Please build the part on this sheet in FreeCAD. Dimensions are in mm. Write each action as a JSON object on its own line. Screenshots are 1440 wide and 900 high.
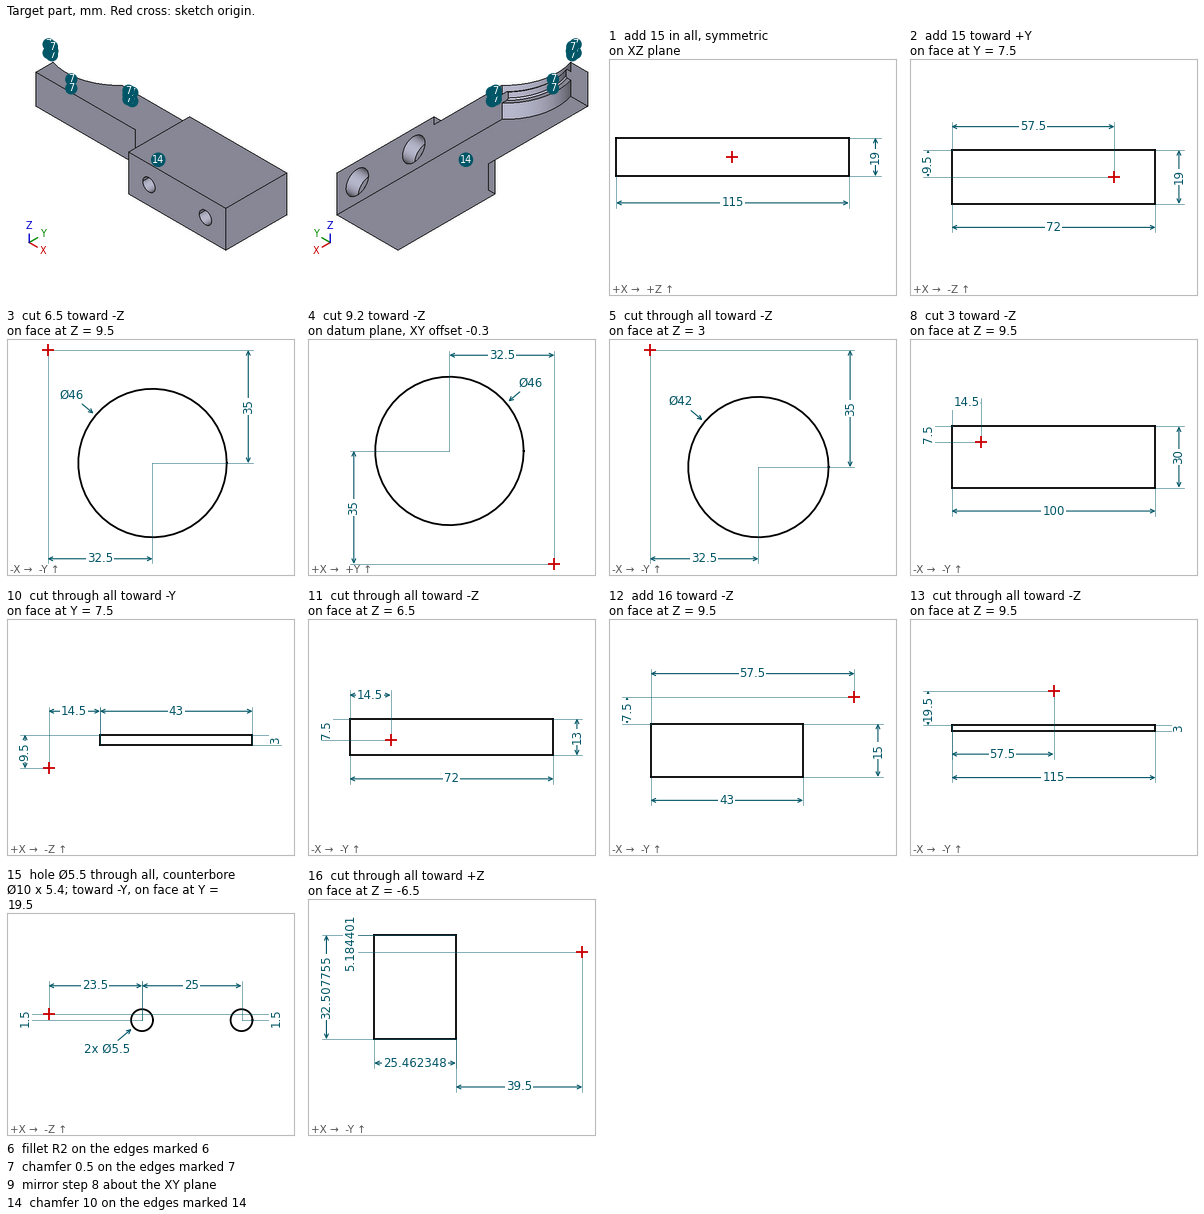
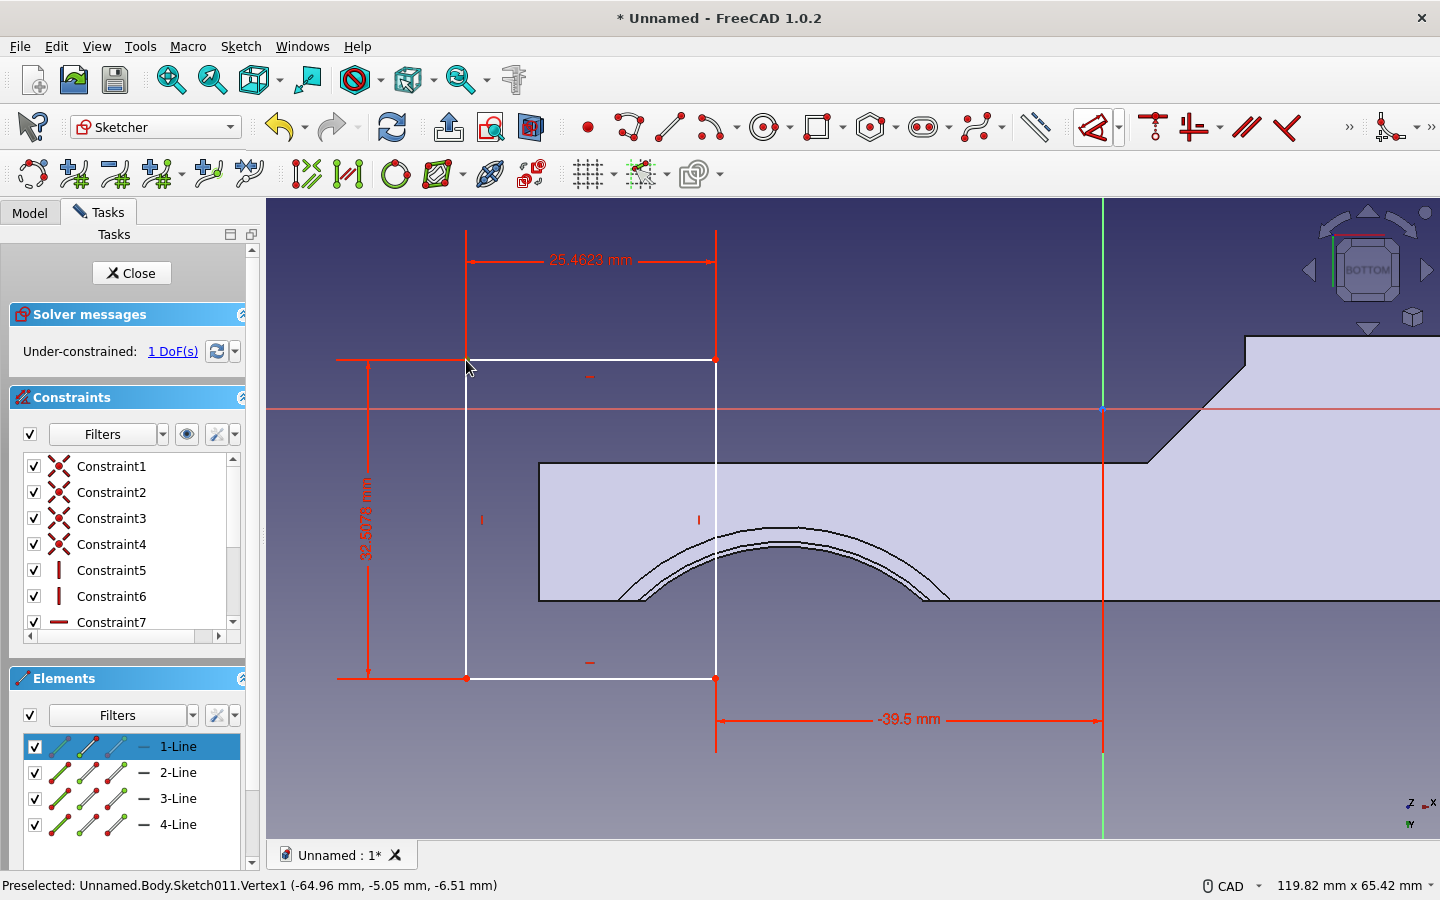
{"action": "left_click", "coordinate": [1118, 128]}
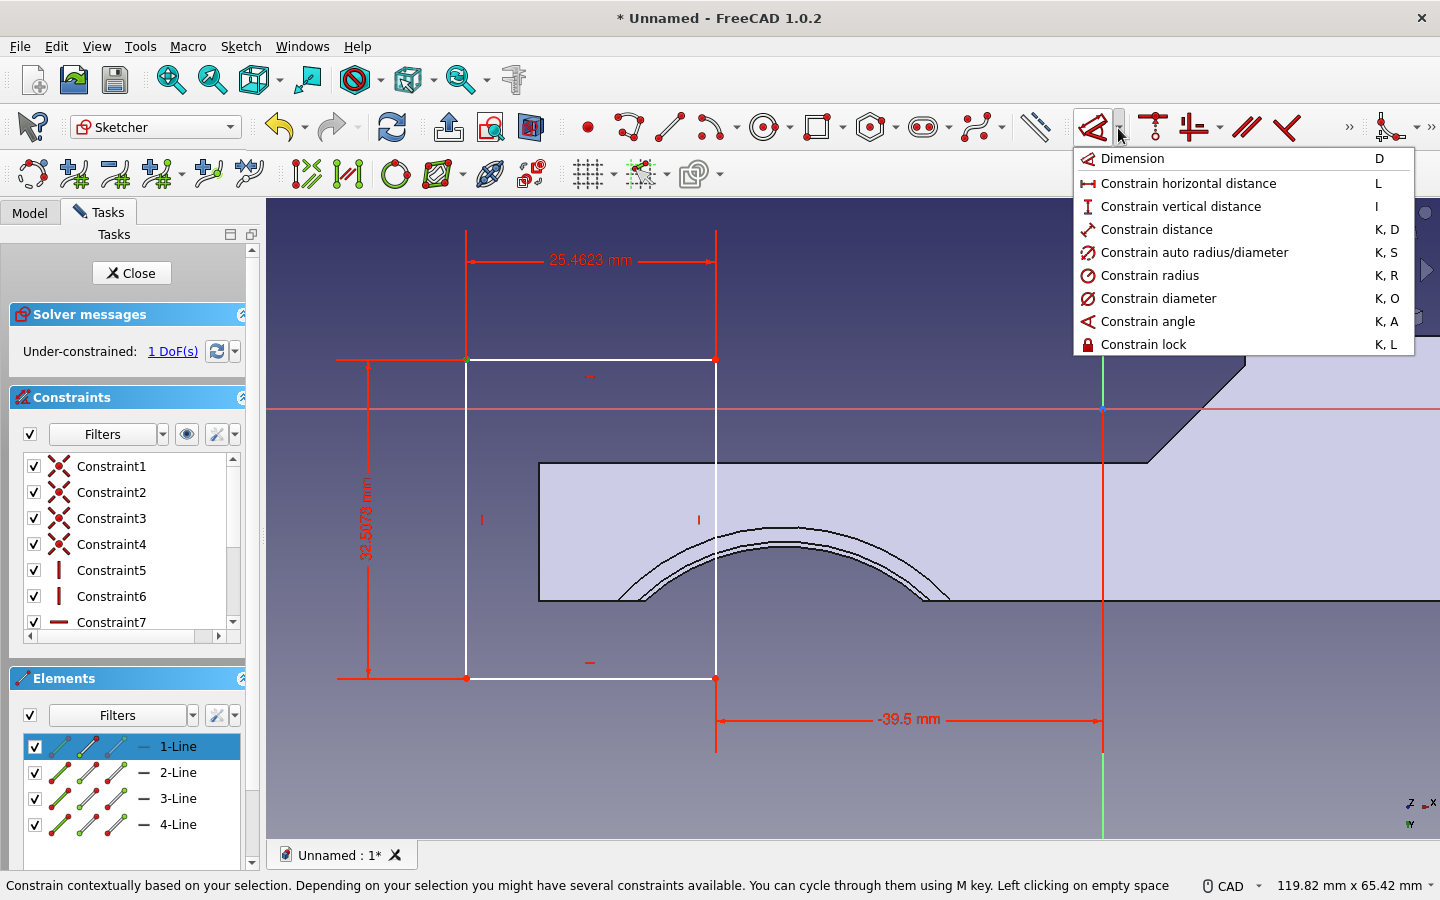
{"action": "left_click", "coordinate": [1244, 206]}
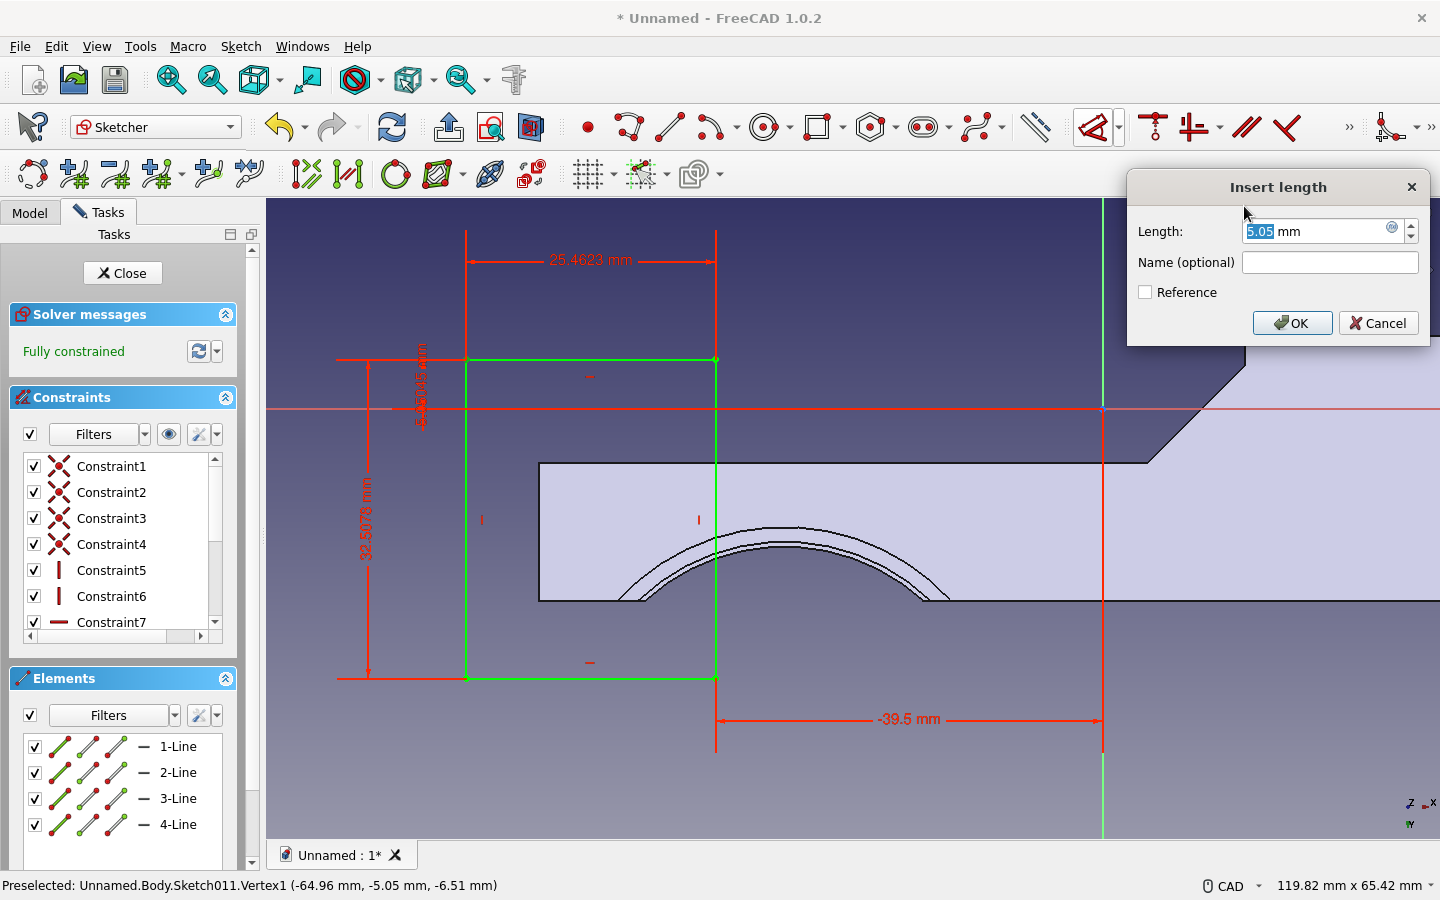
{"action": "type", "text": "5.184401"}
{"action": "key", "text": "Return"}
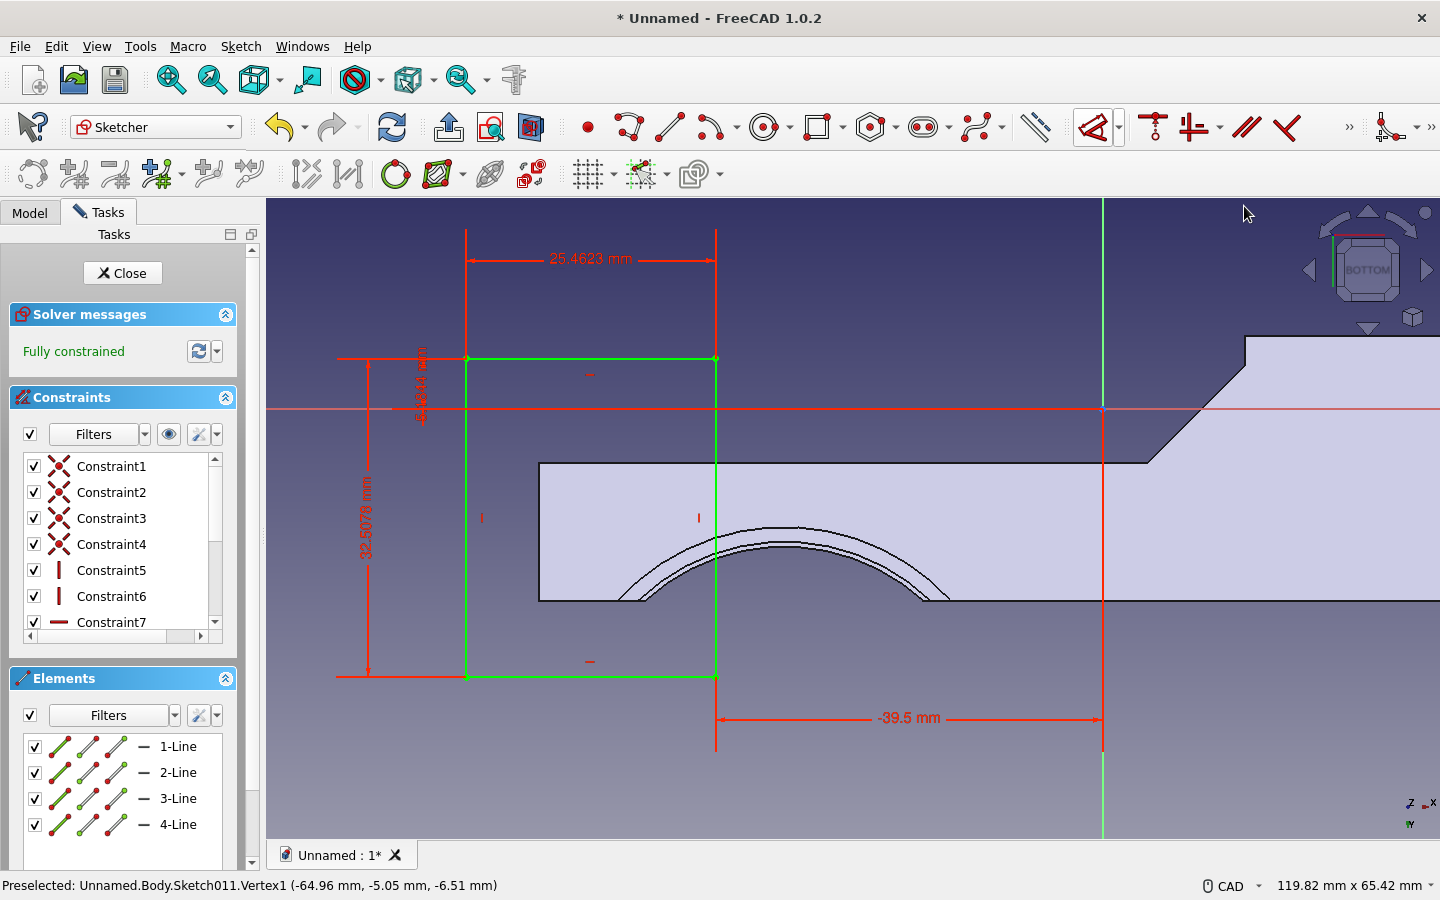
{"action": "left_click", "coordinate": [123, 273]}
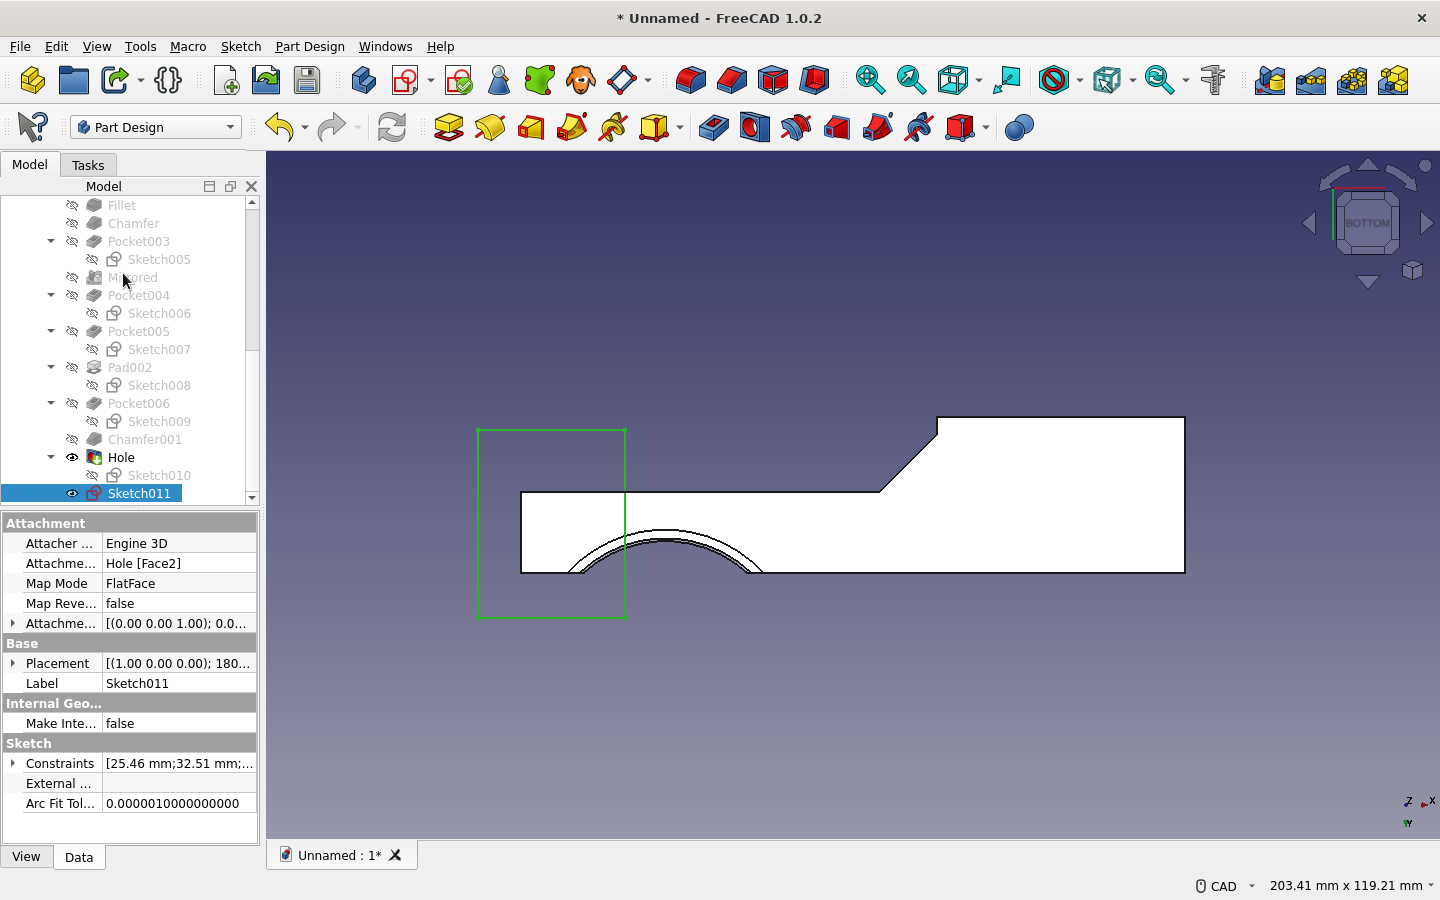
{"action": "left_click", "coordinate": [714, 128]}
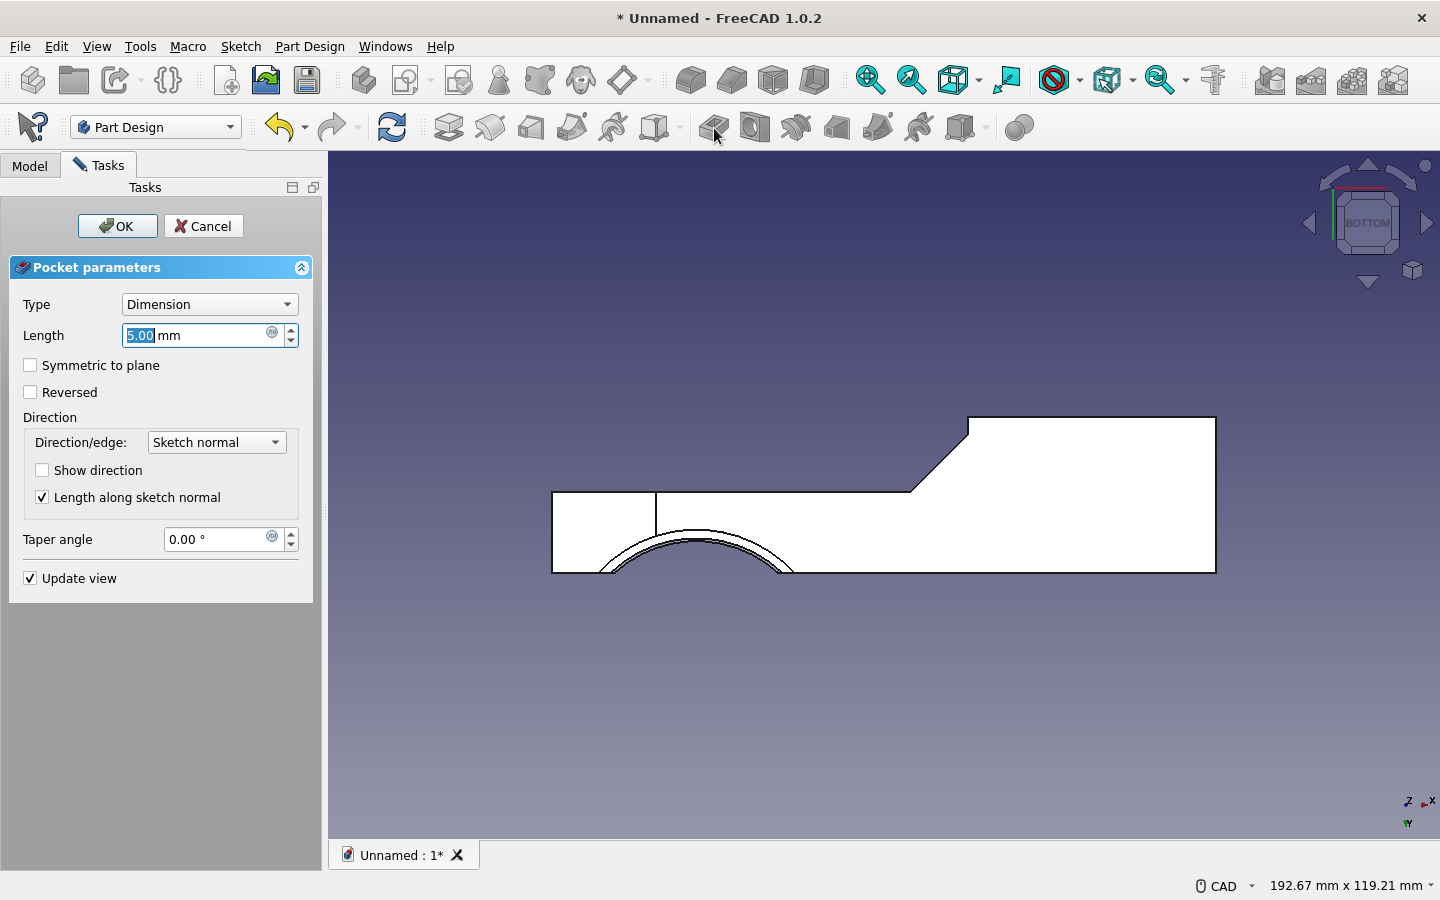
{"action": "left_click", "coordinate": [210, 304]}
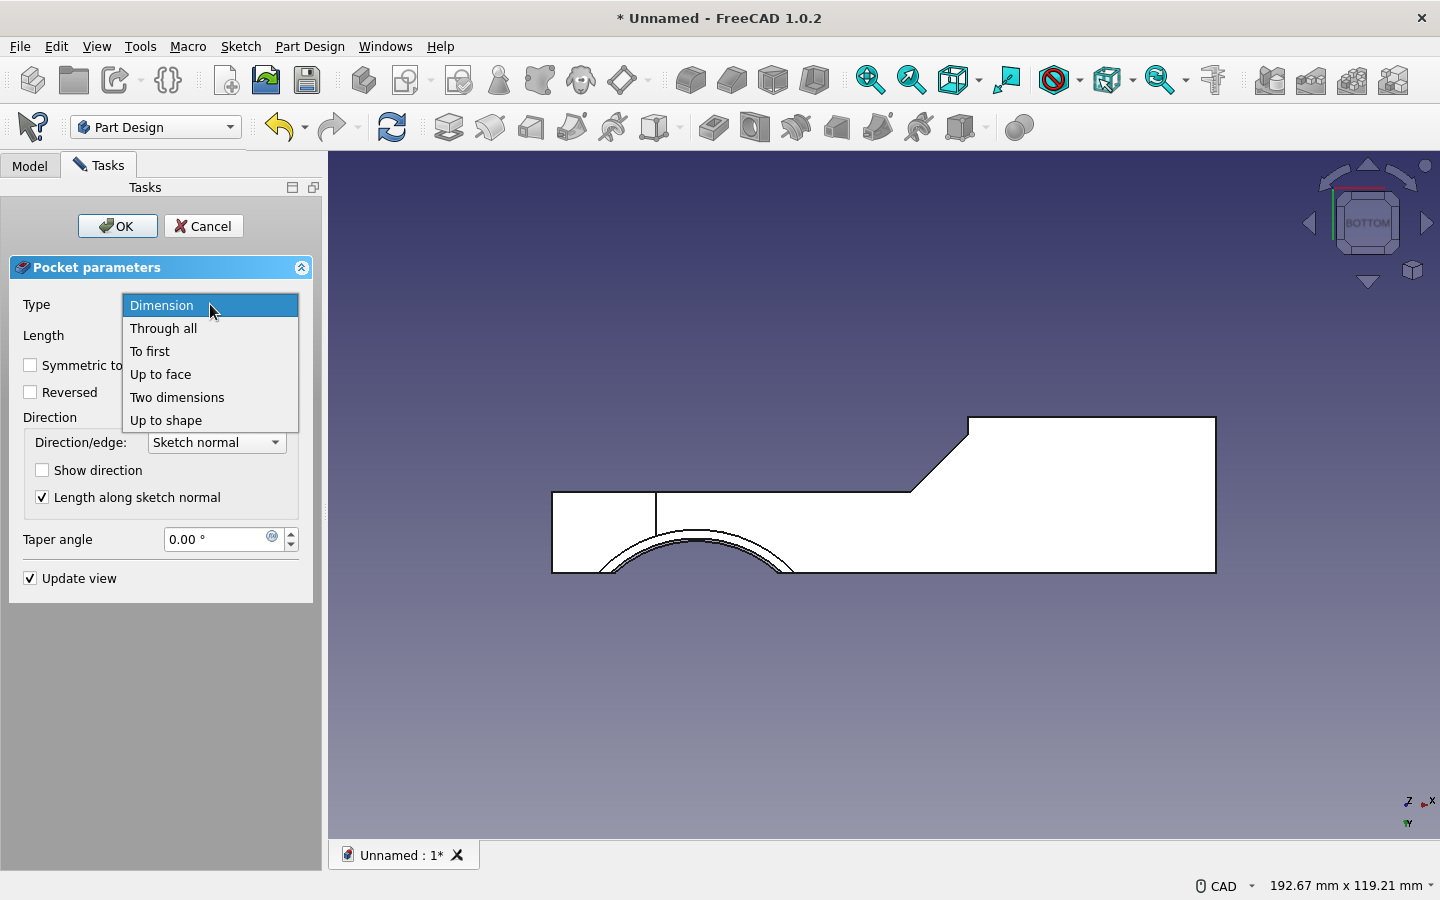
{"action": "left_click", "coordinate": [208, 328]}